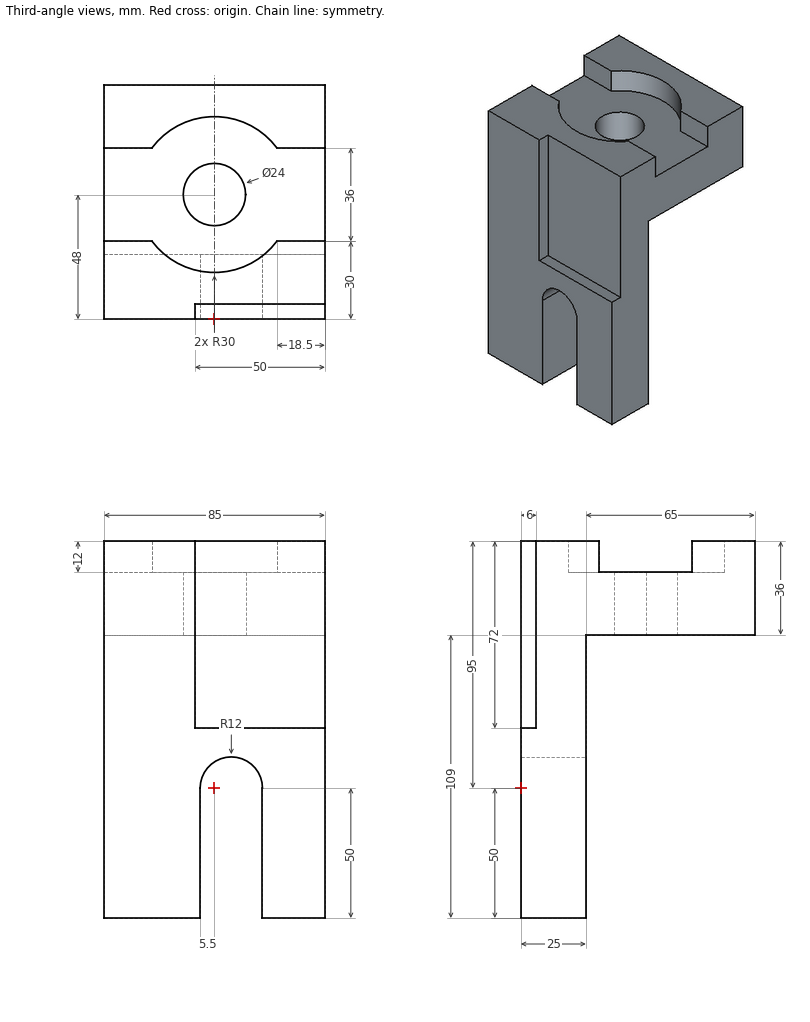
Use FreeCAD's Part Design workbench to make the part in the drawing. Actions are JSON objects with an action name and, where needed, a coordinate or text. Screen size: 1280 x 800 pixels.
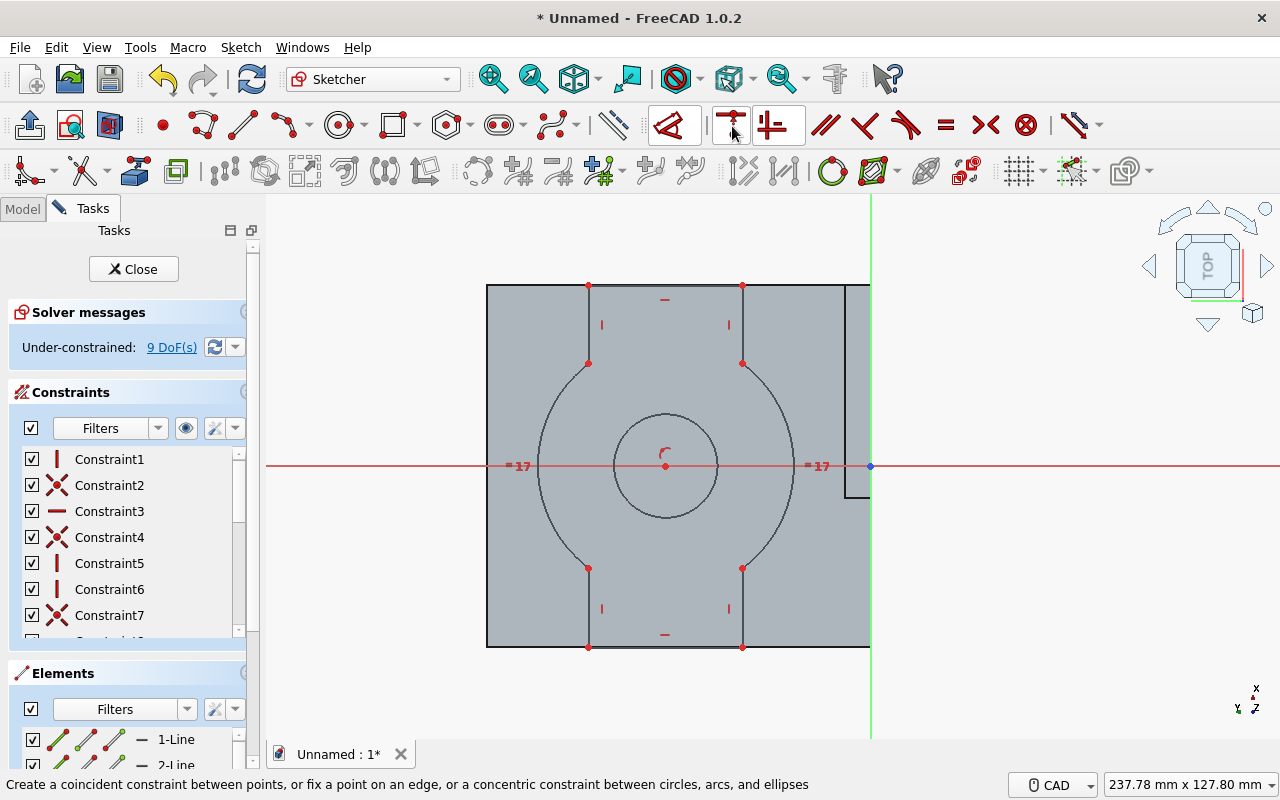
{"action": "left_click", "coordinate": [589, 286]}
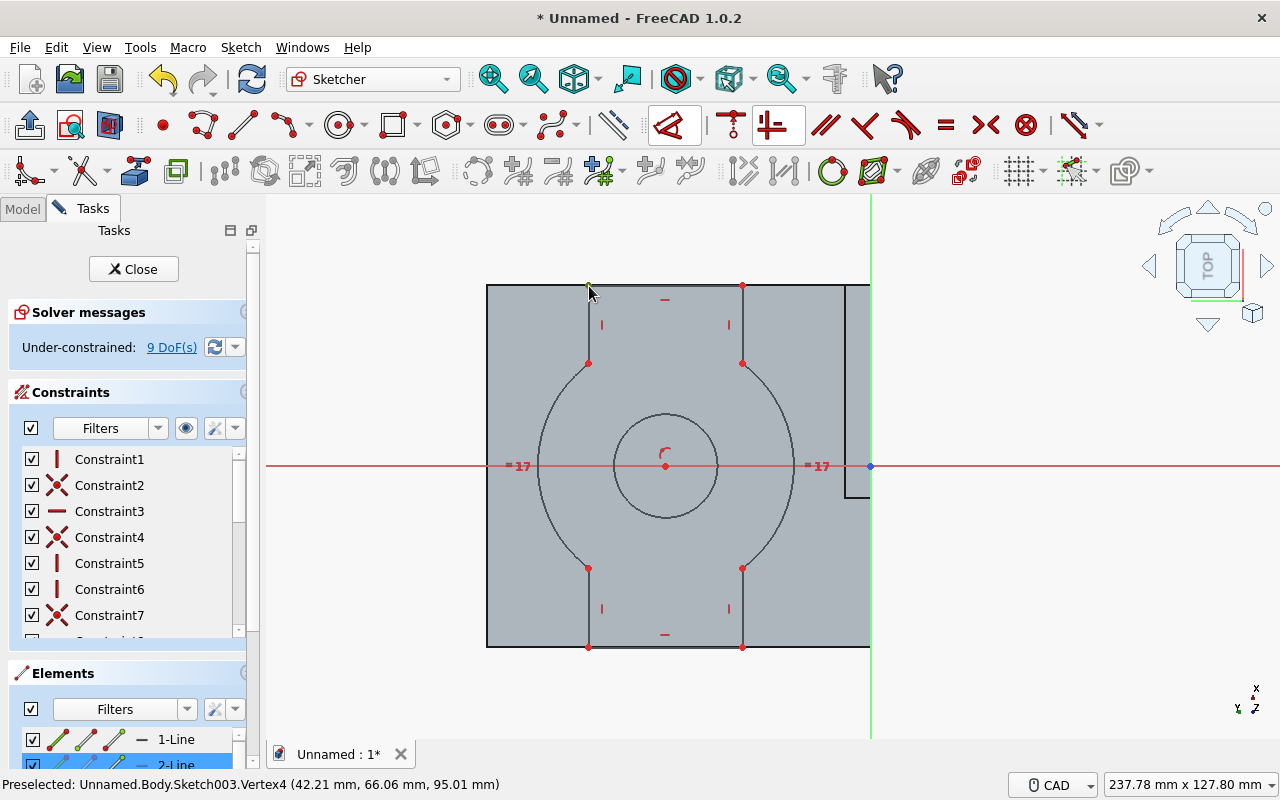
{"action": "left_click", "coordinate": [589, 648]}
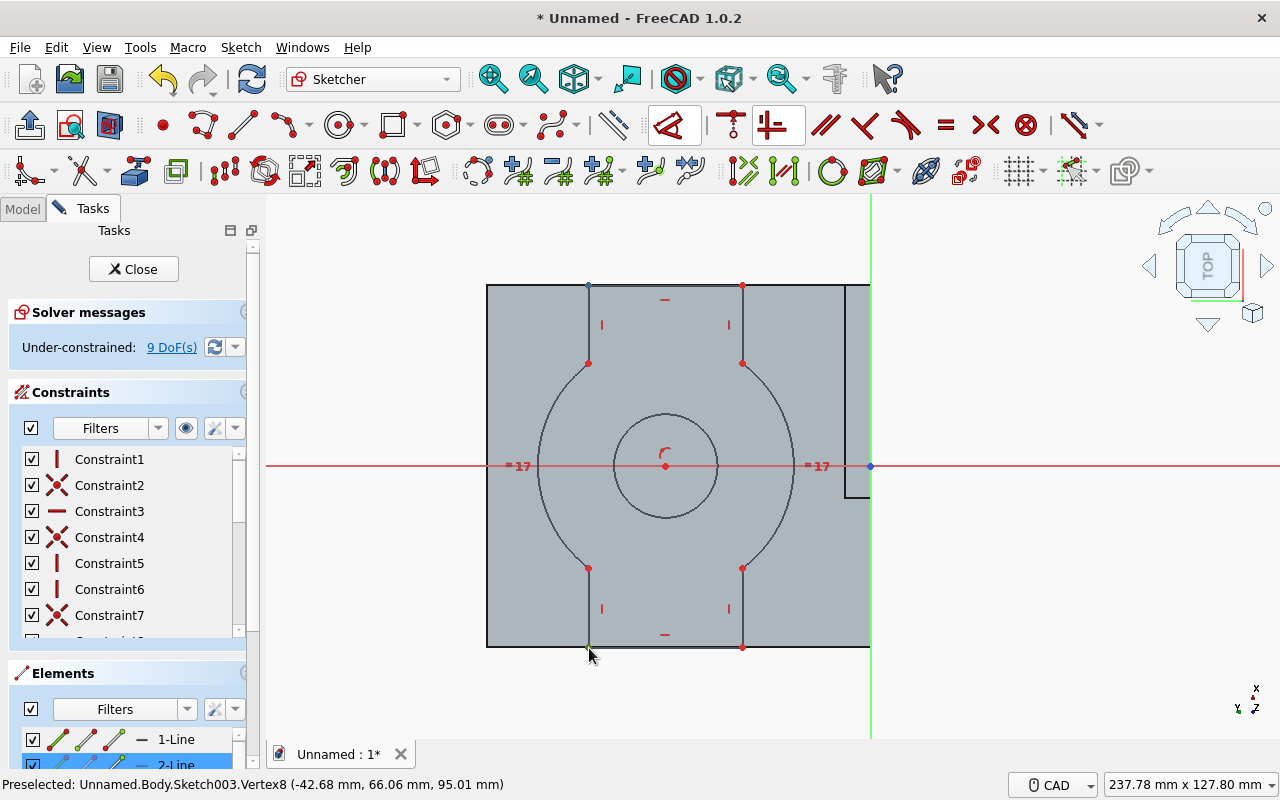
{"action": "left_click", "coordinate": [353, 466]}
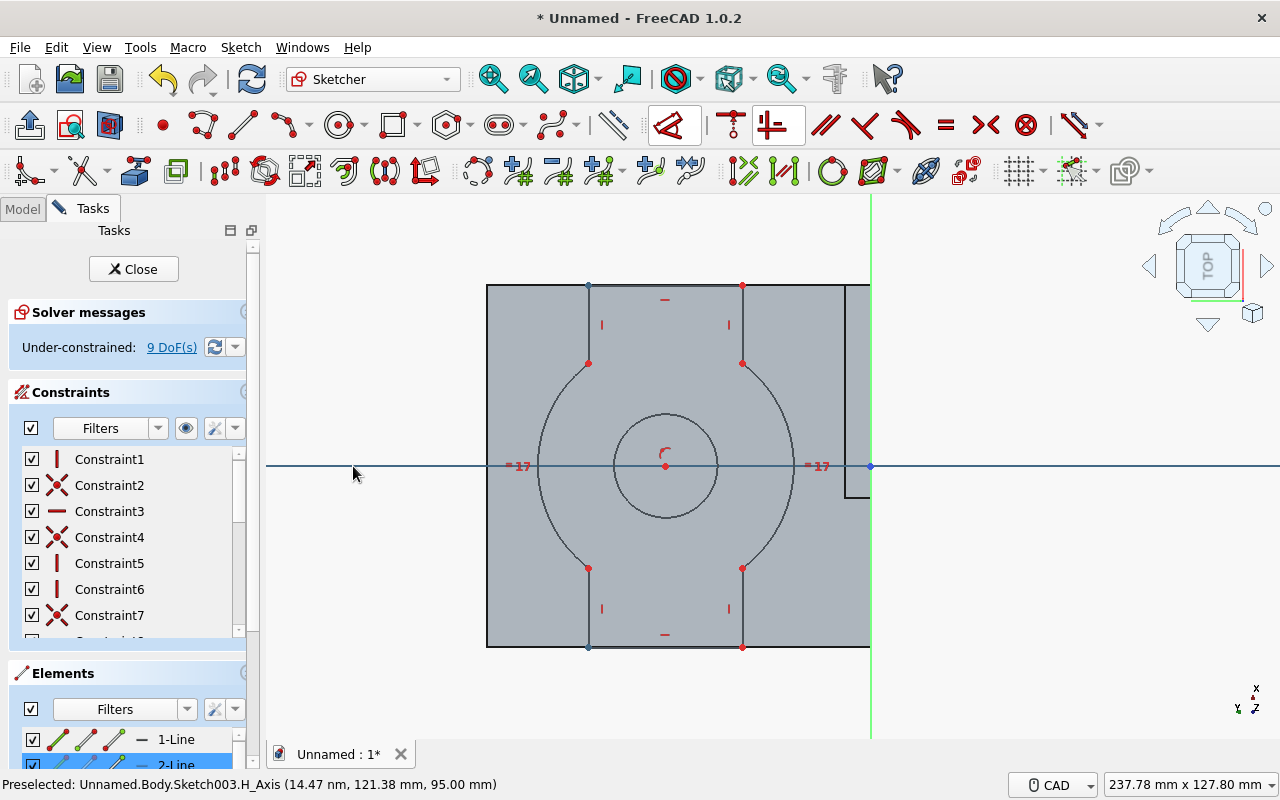
{"action": "left_click", "coordinate": [986, 126]}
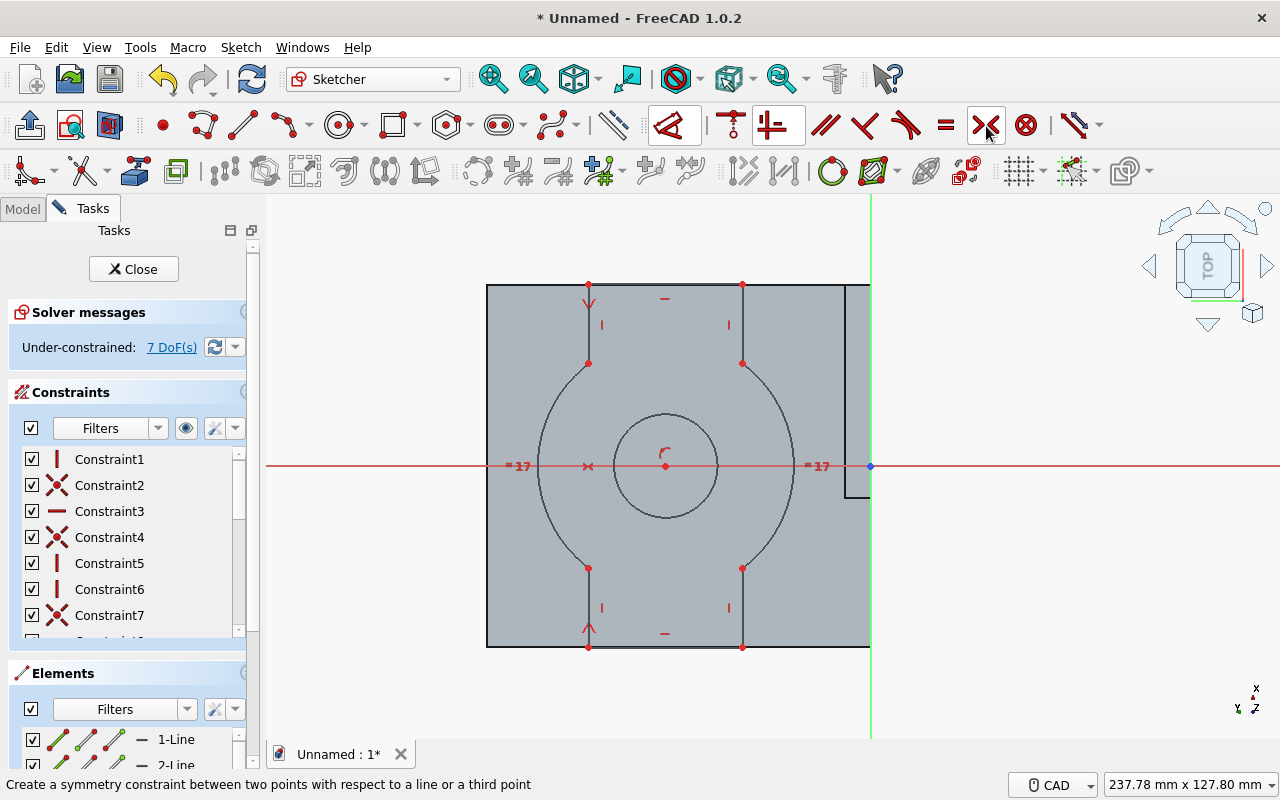
{"action": "left_click", "coordinate": [547, 420]}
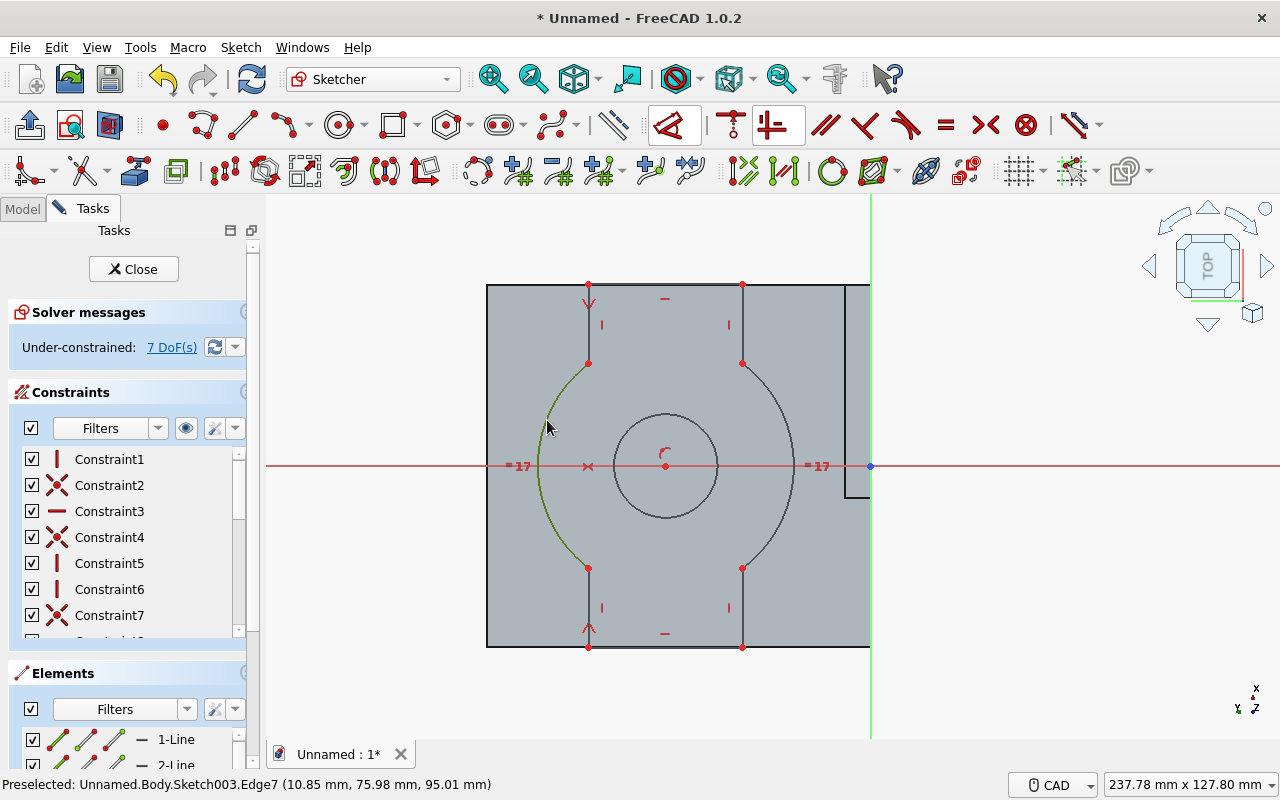
{"action": "key", "text": "k r"}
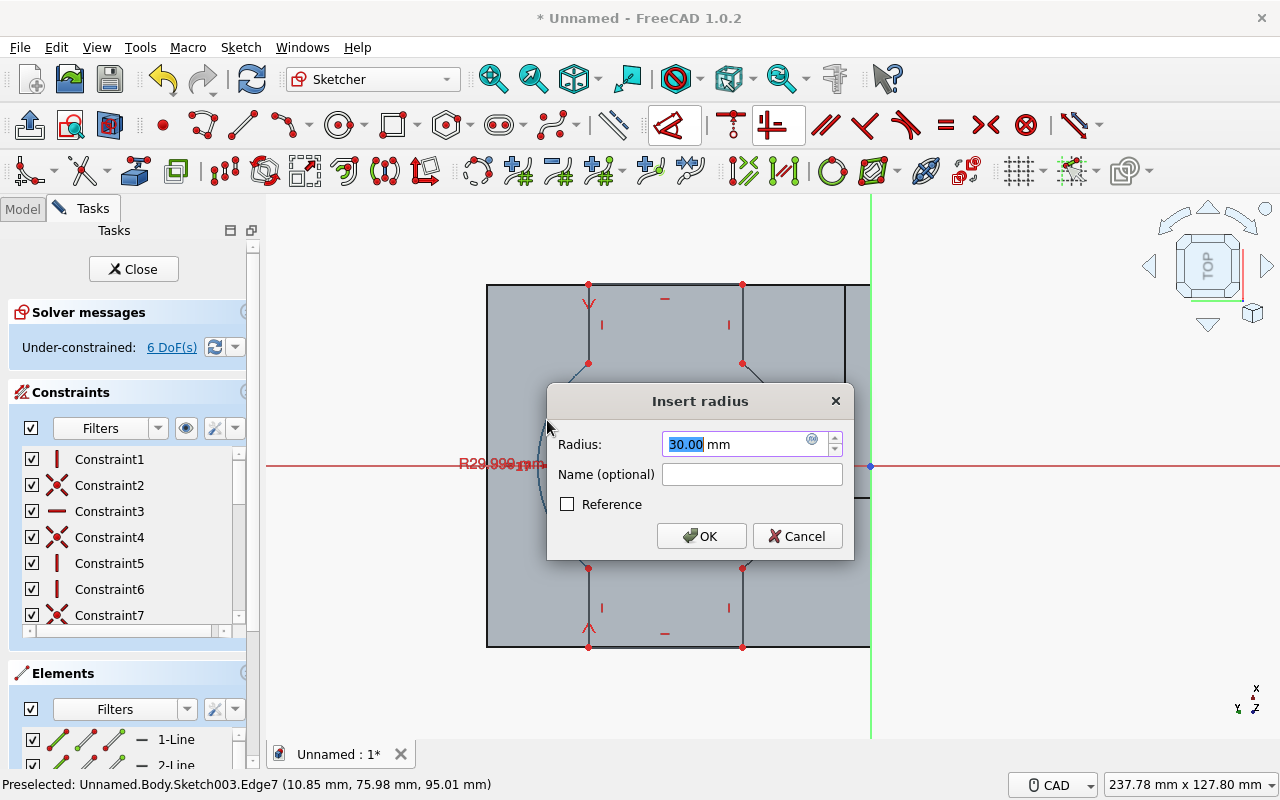
{"action": "type", "text": "30"}
{"action": "key", "text": "Return"}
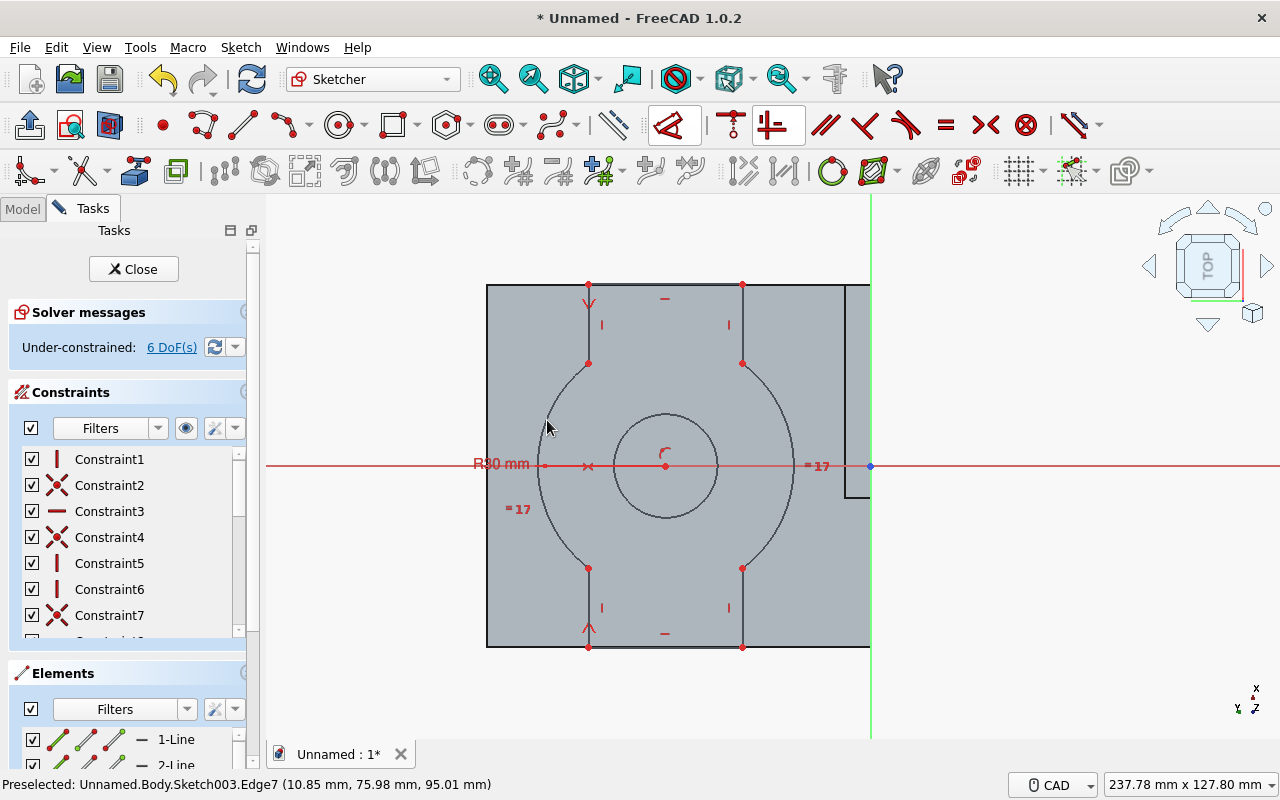
{"action": "left_click", "coordinate": [702, 429]}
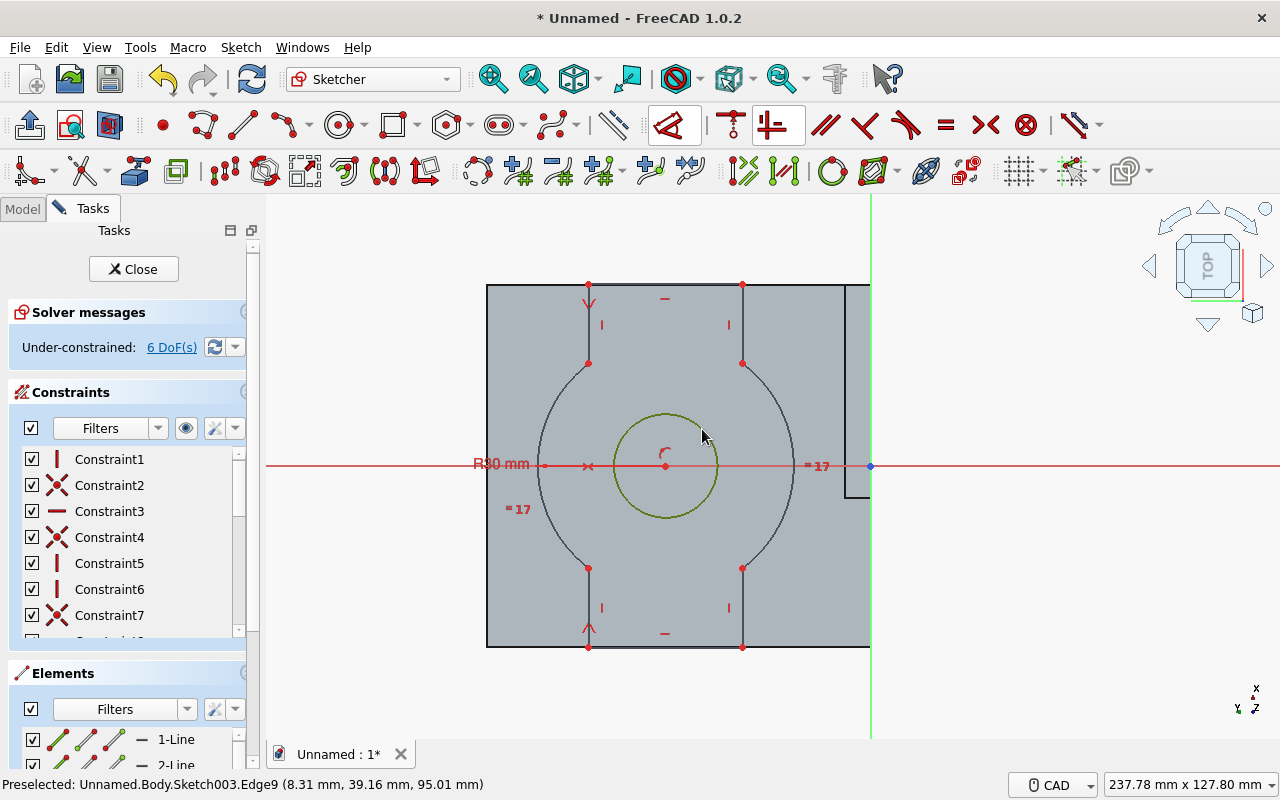
{"action": "left_click", "coordinate": [696, 126]}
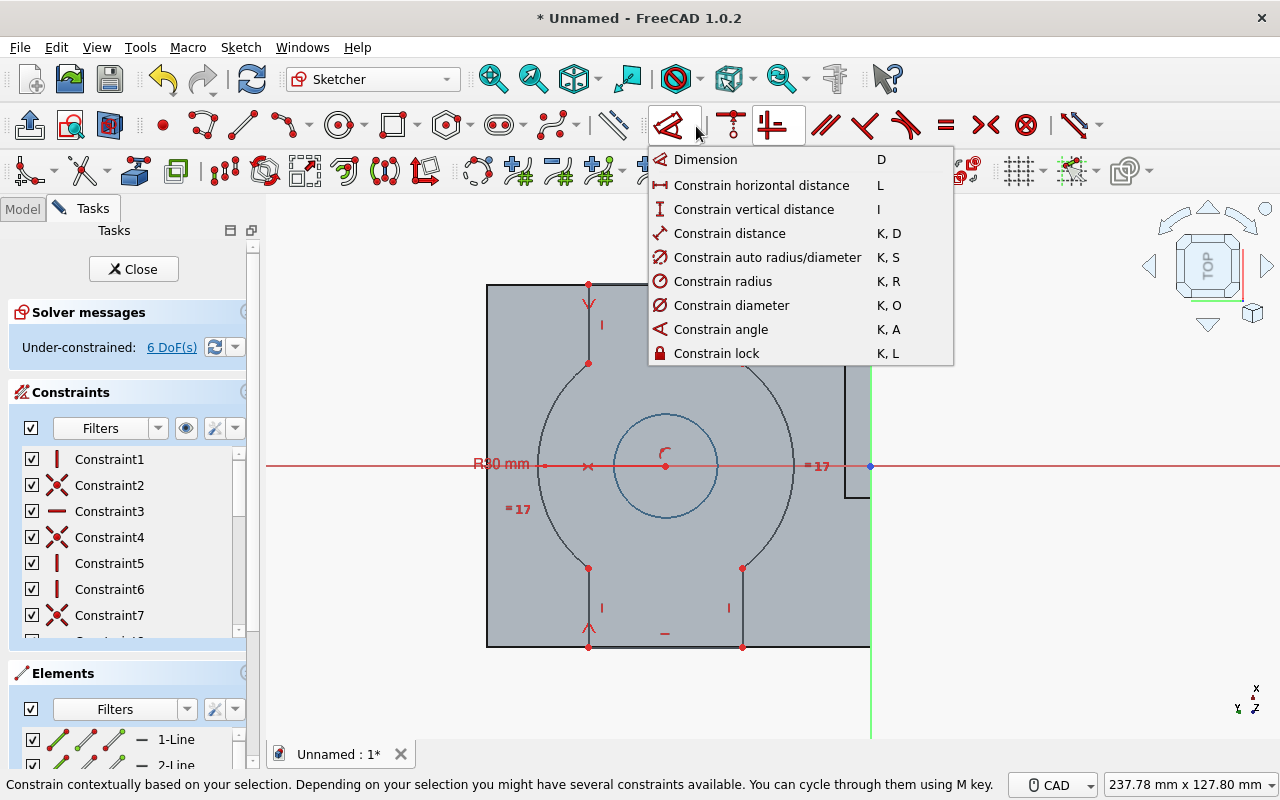
{"action": "left_click", "coordinate": [801, 305]}